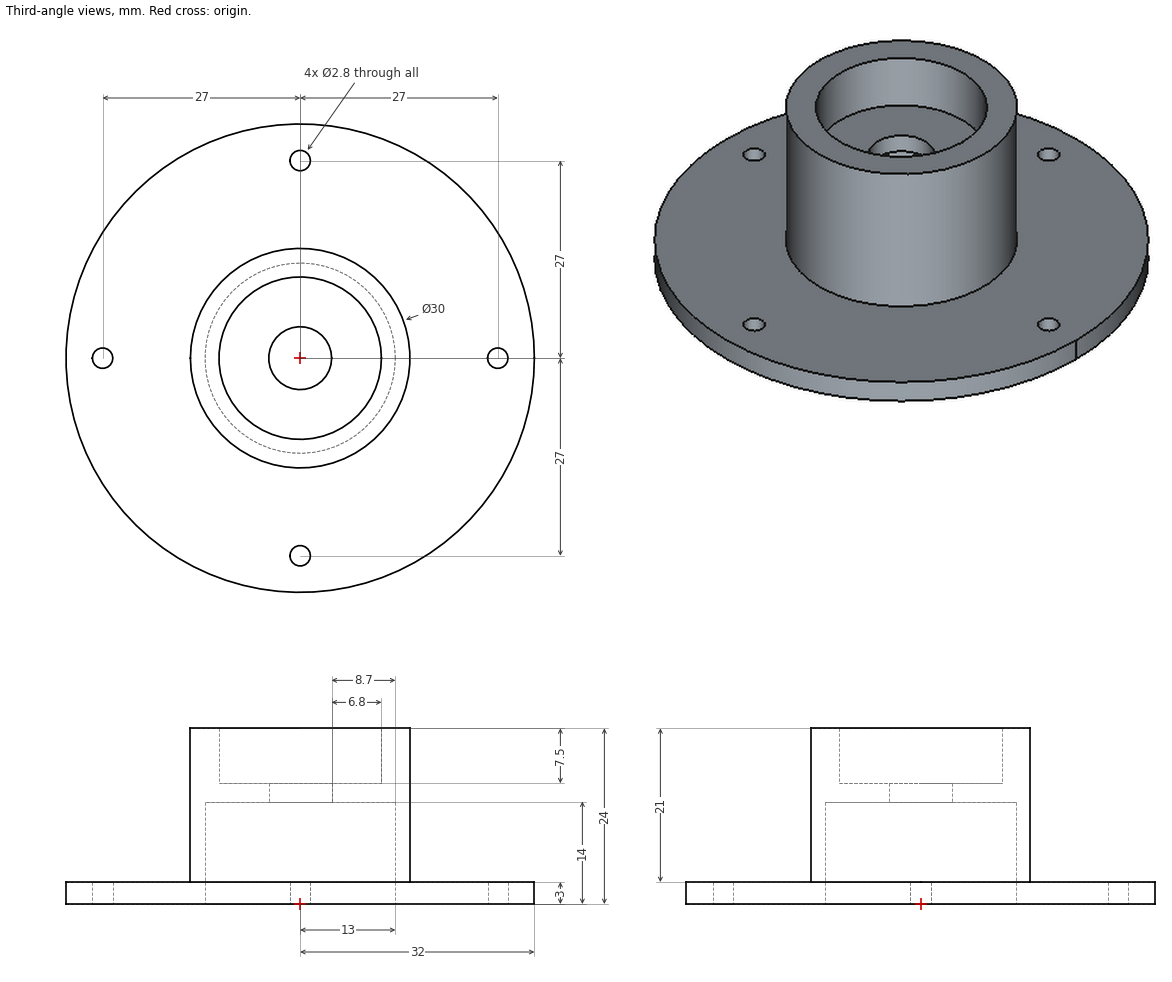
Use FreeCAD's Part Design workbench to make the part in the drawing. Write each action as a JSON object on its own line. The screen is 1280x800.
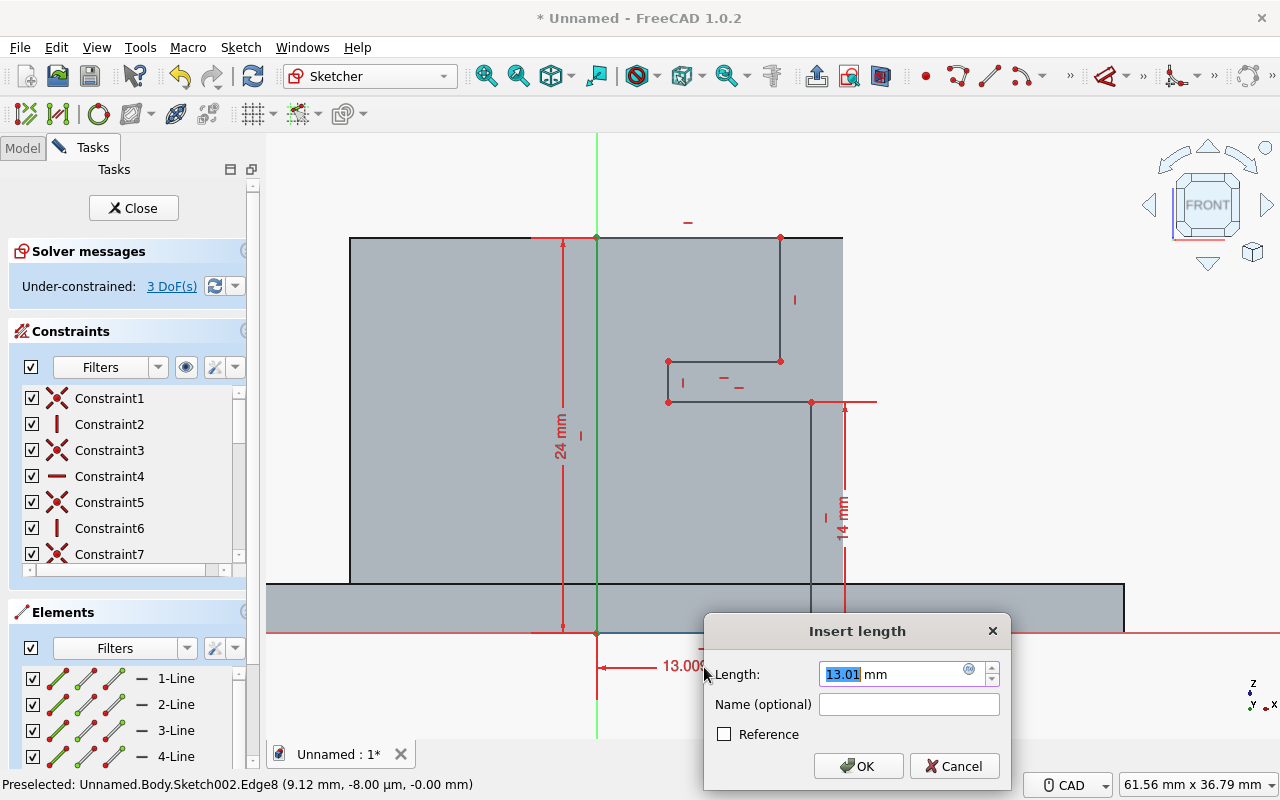
{"action": "type", "text": "13"}
{"action": "key", "text": "Return"}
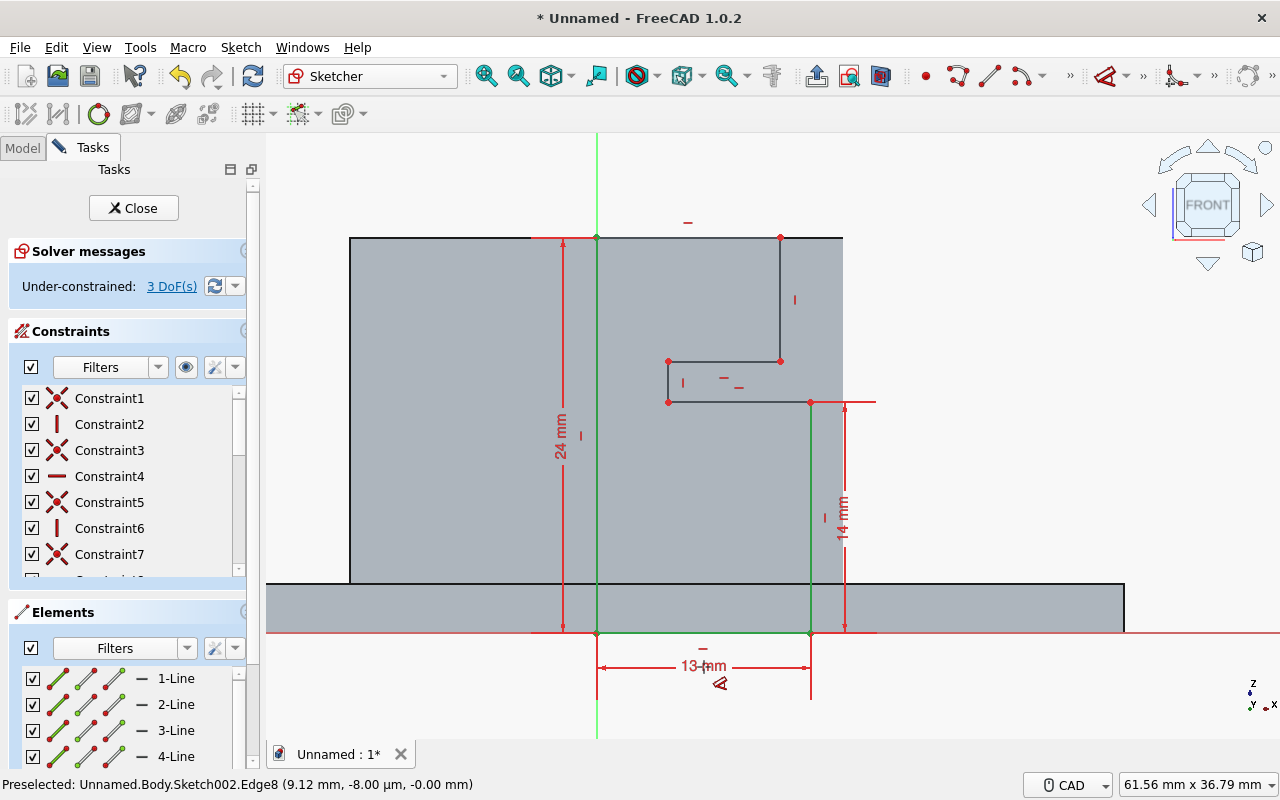
{"action": "left_click", "coordinate": [780, 275]}
{"action": "left_click", "coordinate": [814, 300]}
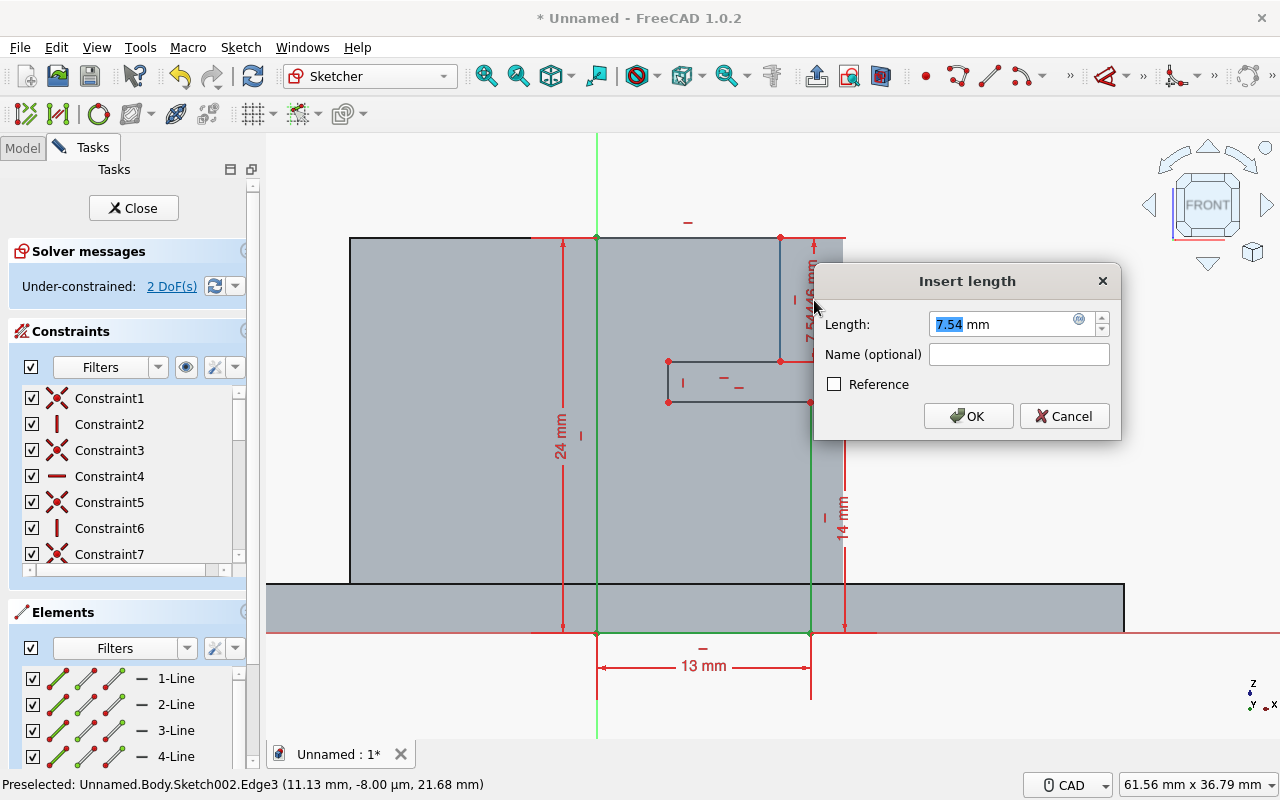
{"action": "type", "text": "7.5"}
{"action": "key", "text": "Return"}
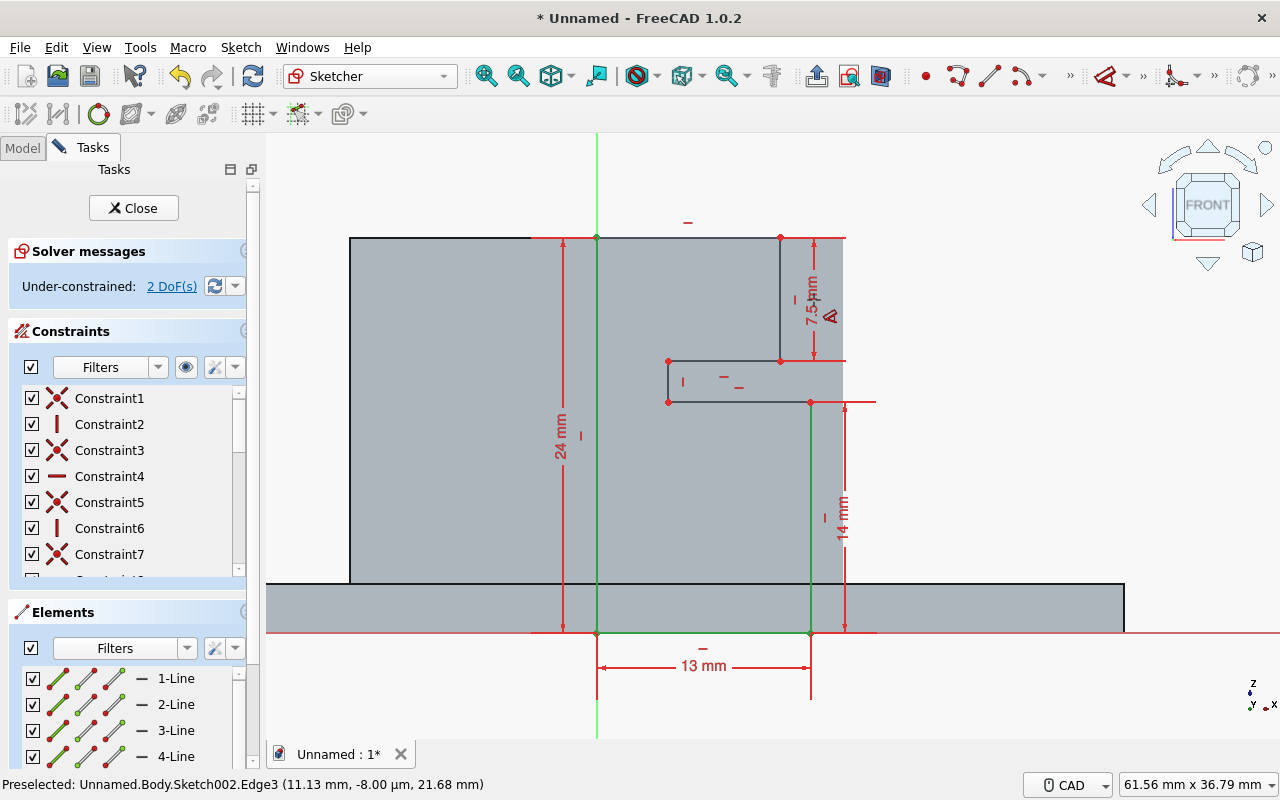
{"action": "left_click", "coordinate": [746, 361]}
{"action": "left_click", "coordinate": [724, 327]}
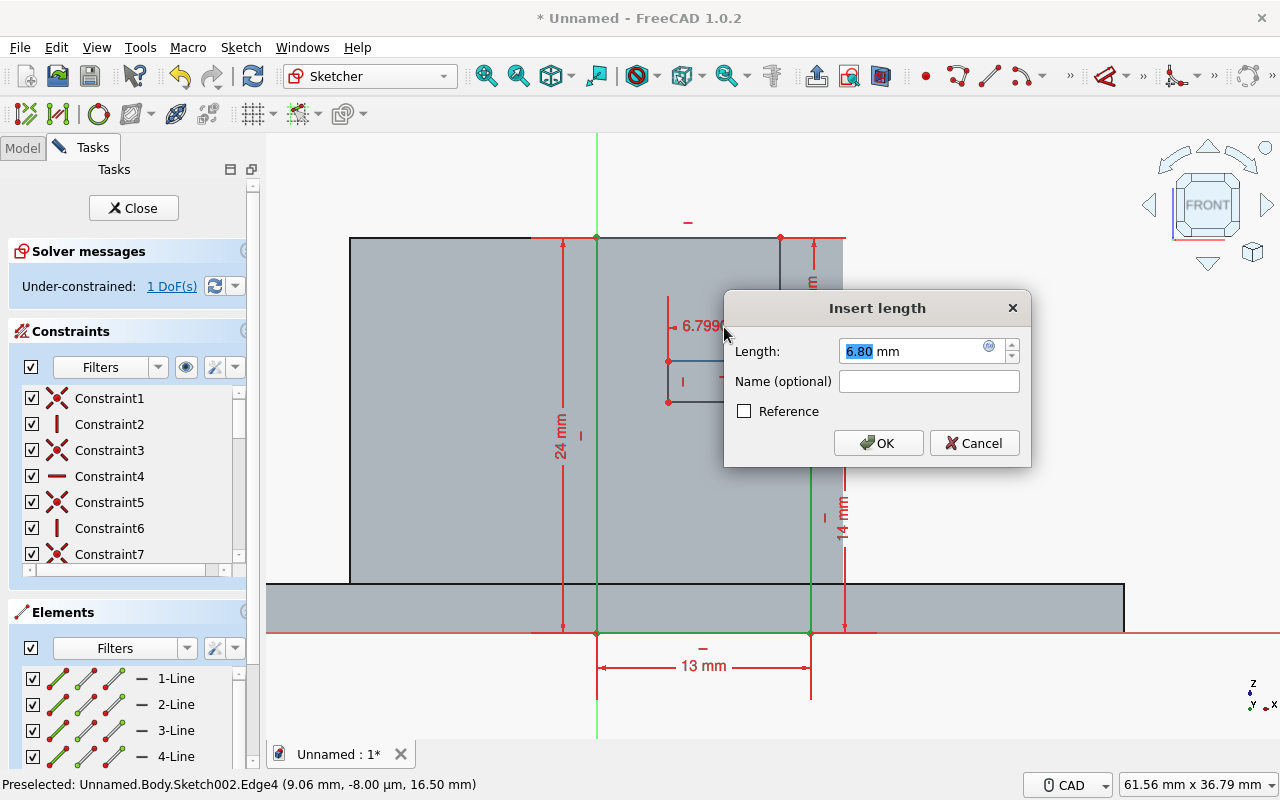
{"action": "type", "text": "6.8"}
{"action": "key", "text": "Return"}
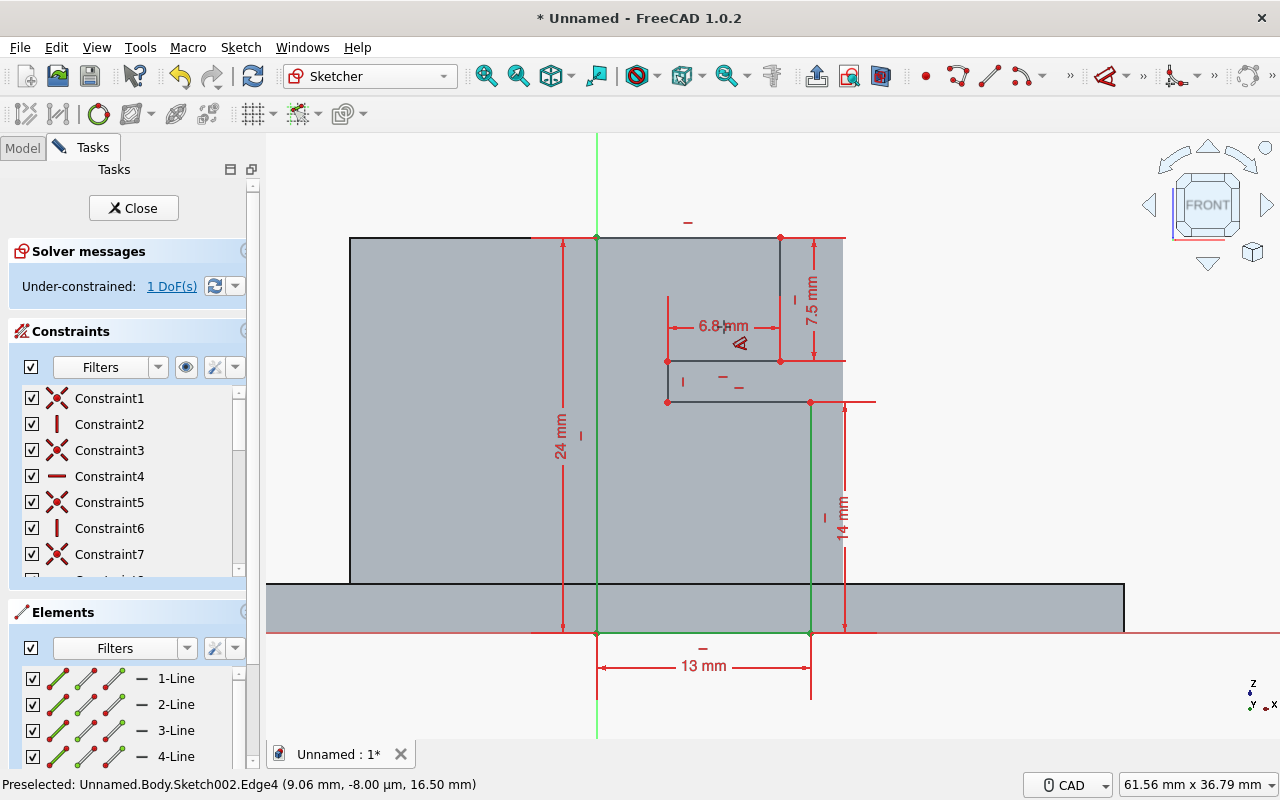
{"action": "left_click", "coordinate": [711, 402]}
{"action": "left_click", "coordinate": [739, 436]}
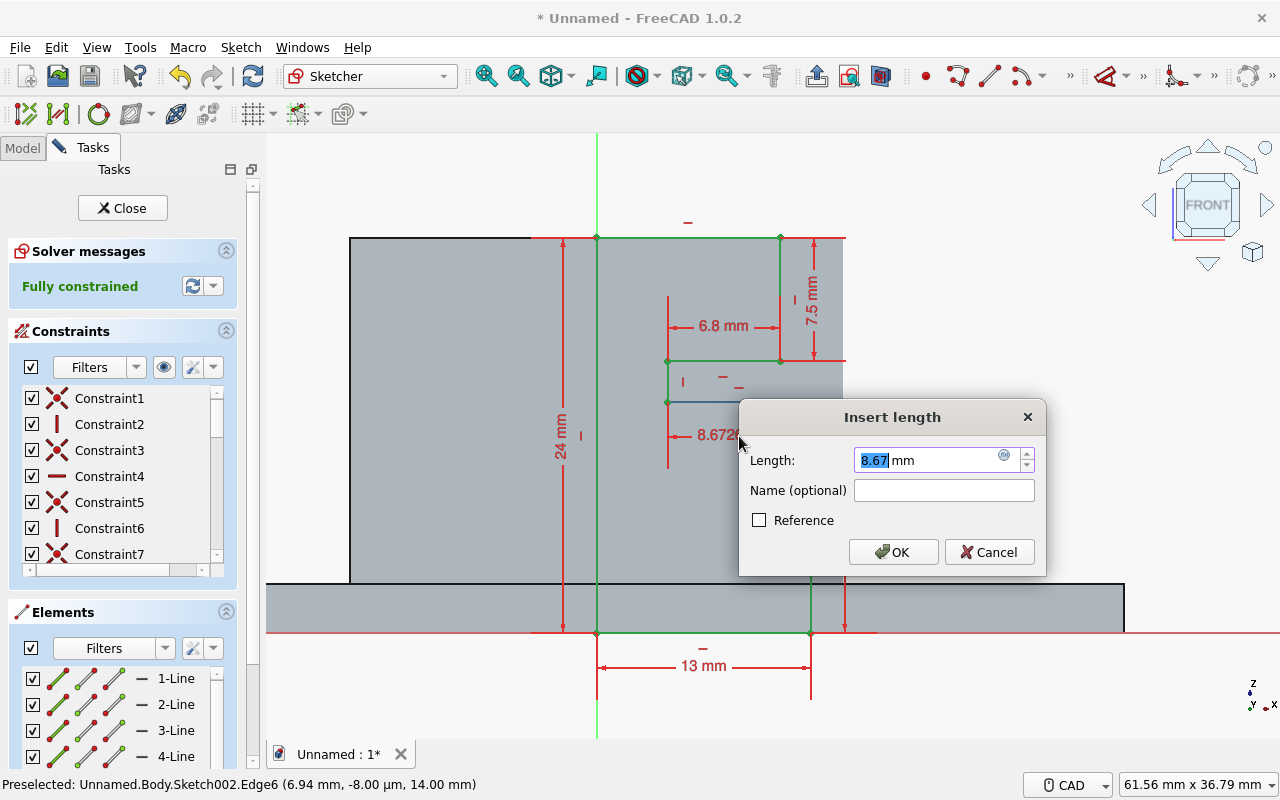
{"action": "type", "text": "8.7"}
{"action": "key", "text": "Return"}
{"action": "key", "text": "Escape"}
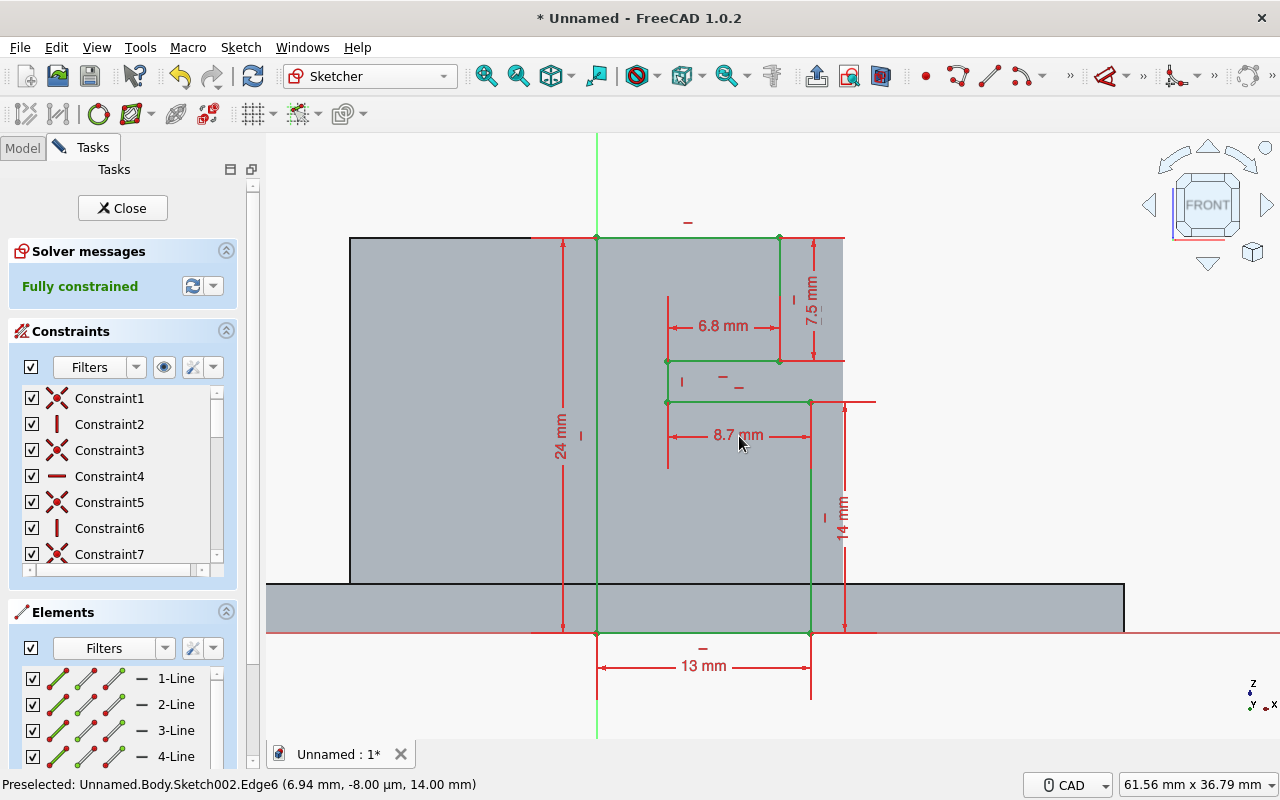
{"action": "left_click", "coordinate": [123, 208]}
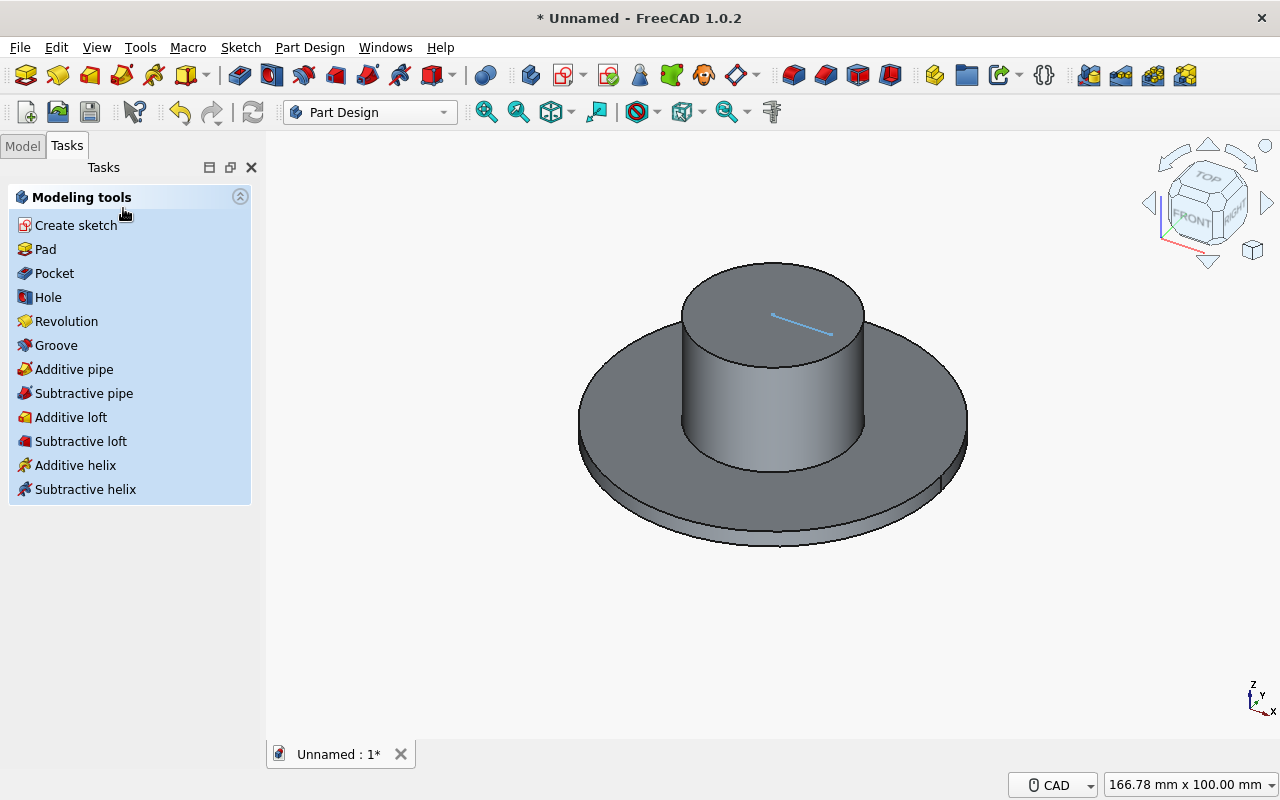
{"action": "left_click", "coordinate": [304, 76]}